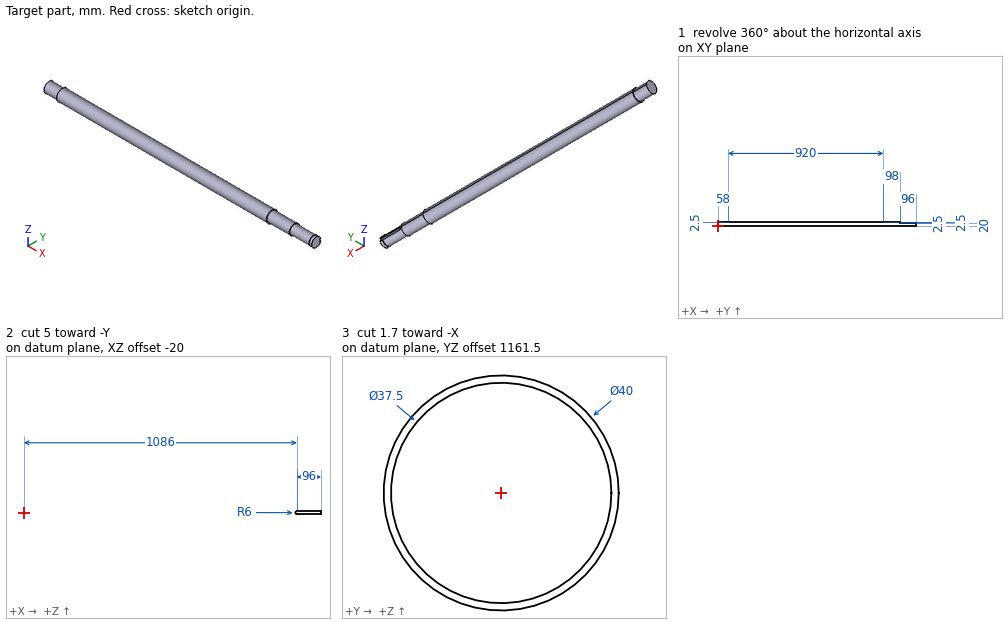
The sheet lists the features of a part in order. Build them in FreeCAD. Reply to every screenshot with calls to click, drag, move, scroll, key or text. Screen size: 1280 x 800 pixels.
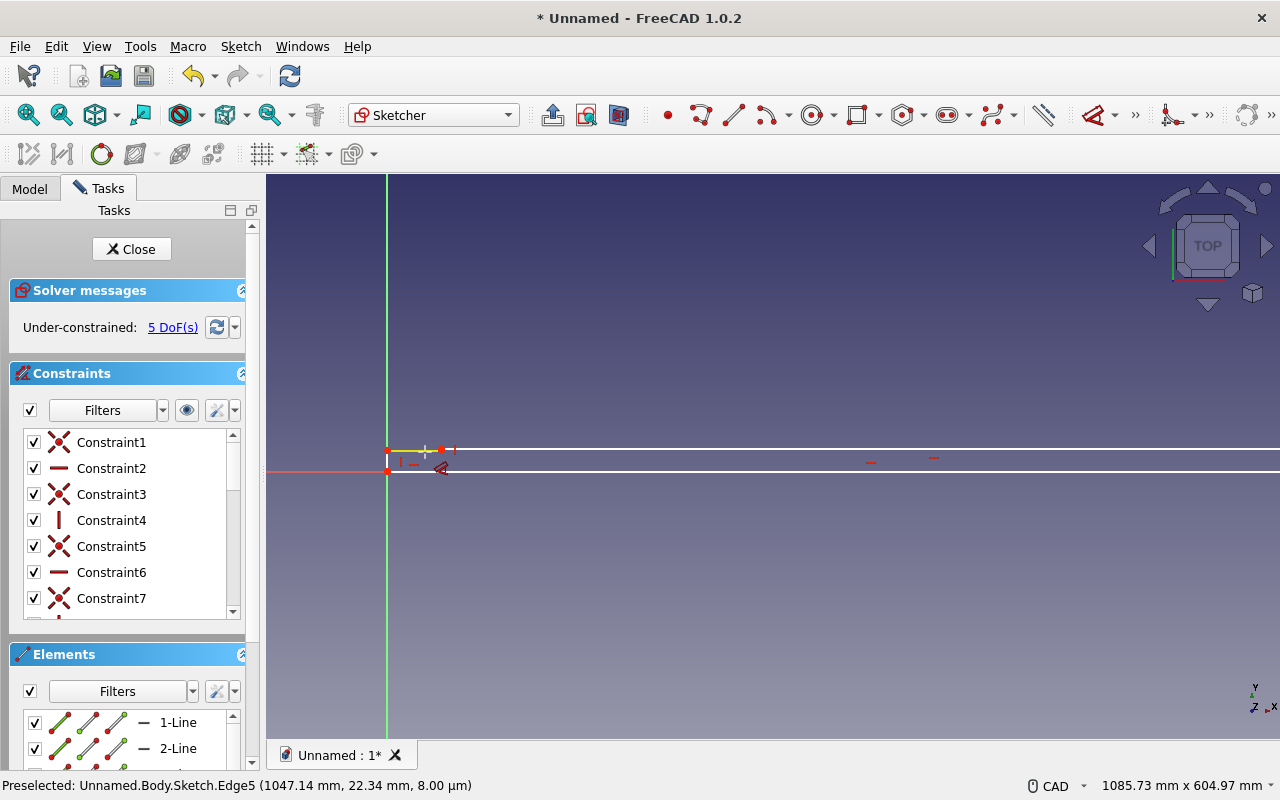
click(425, 451)
click(414, 417)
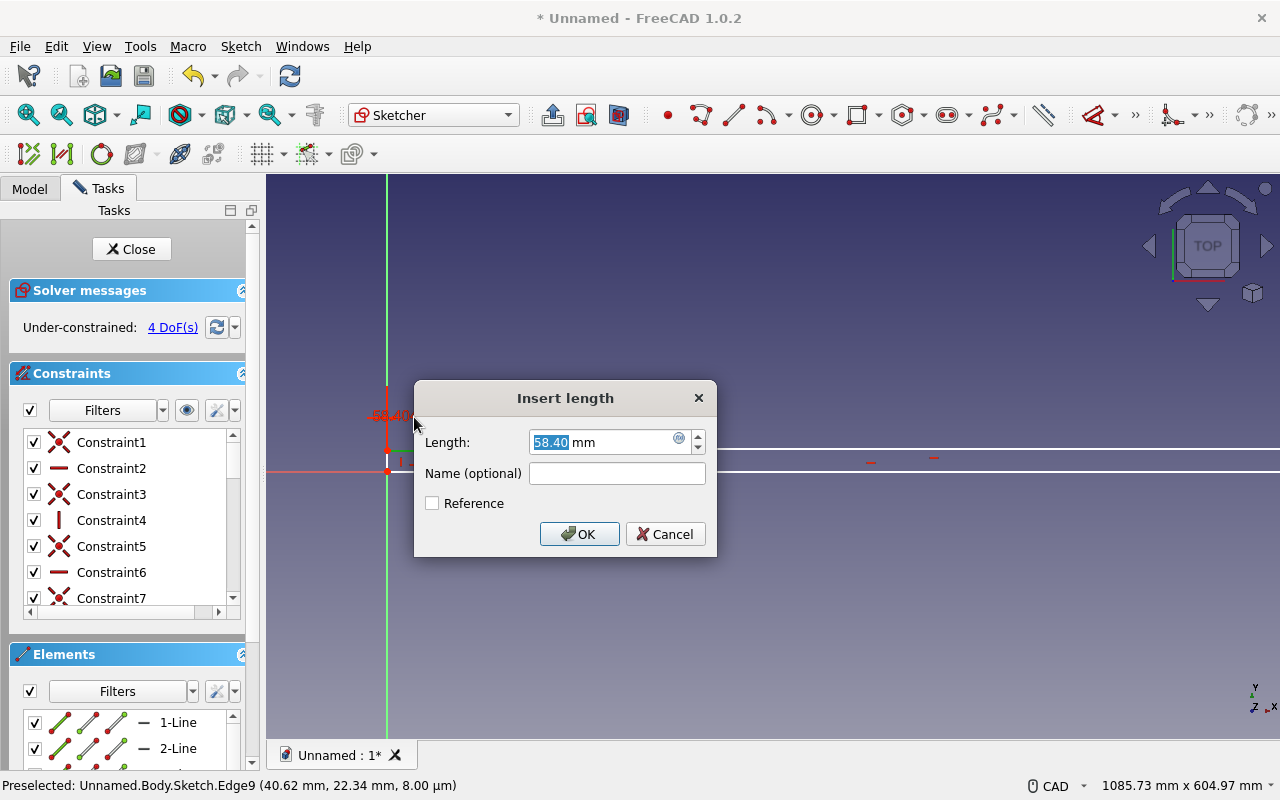
text(58)
key(Return)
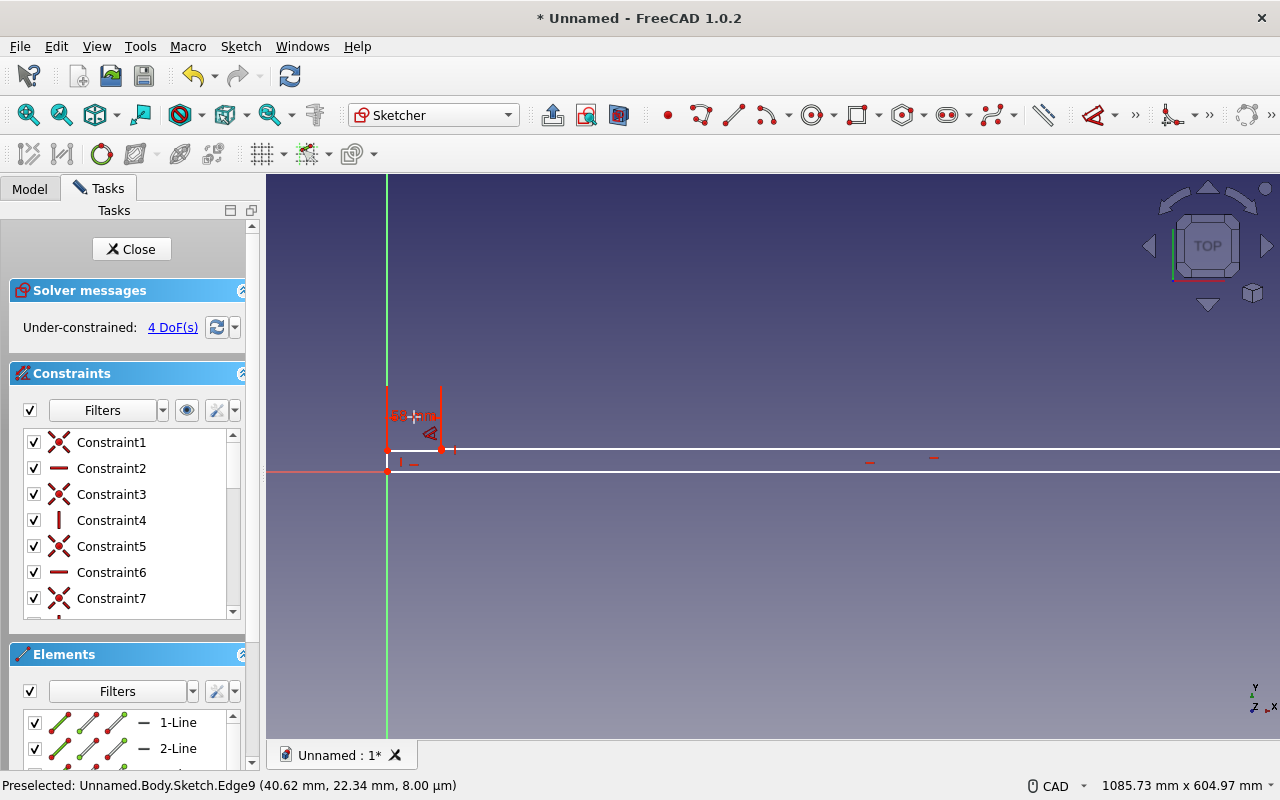
scroll(425, 452, down, 3)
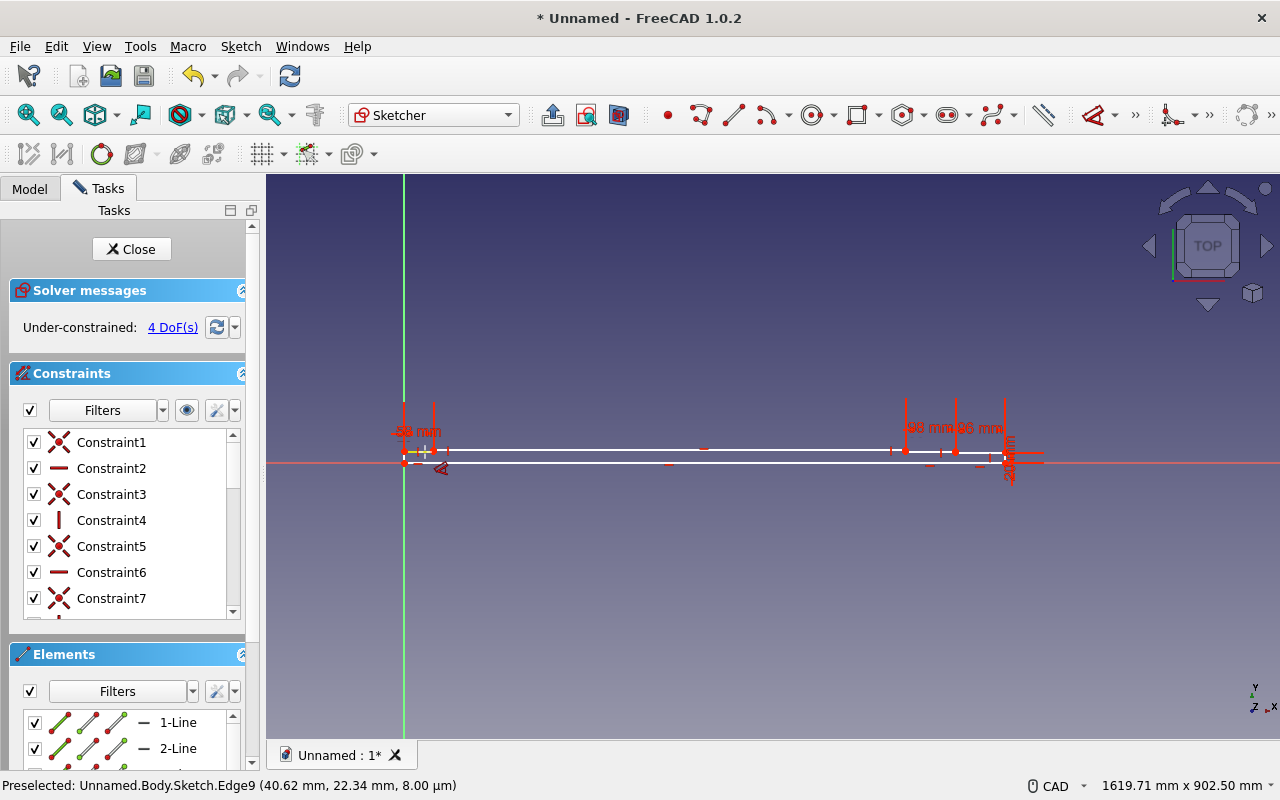
scroll(956, 452, up, 18)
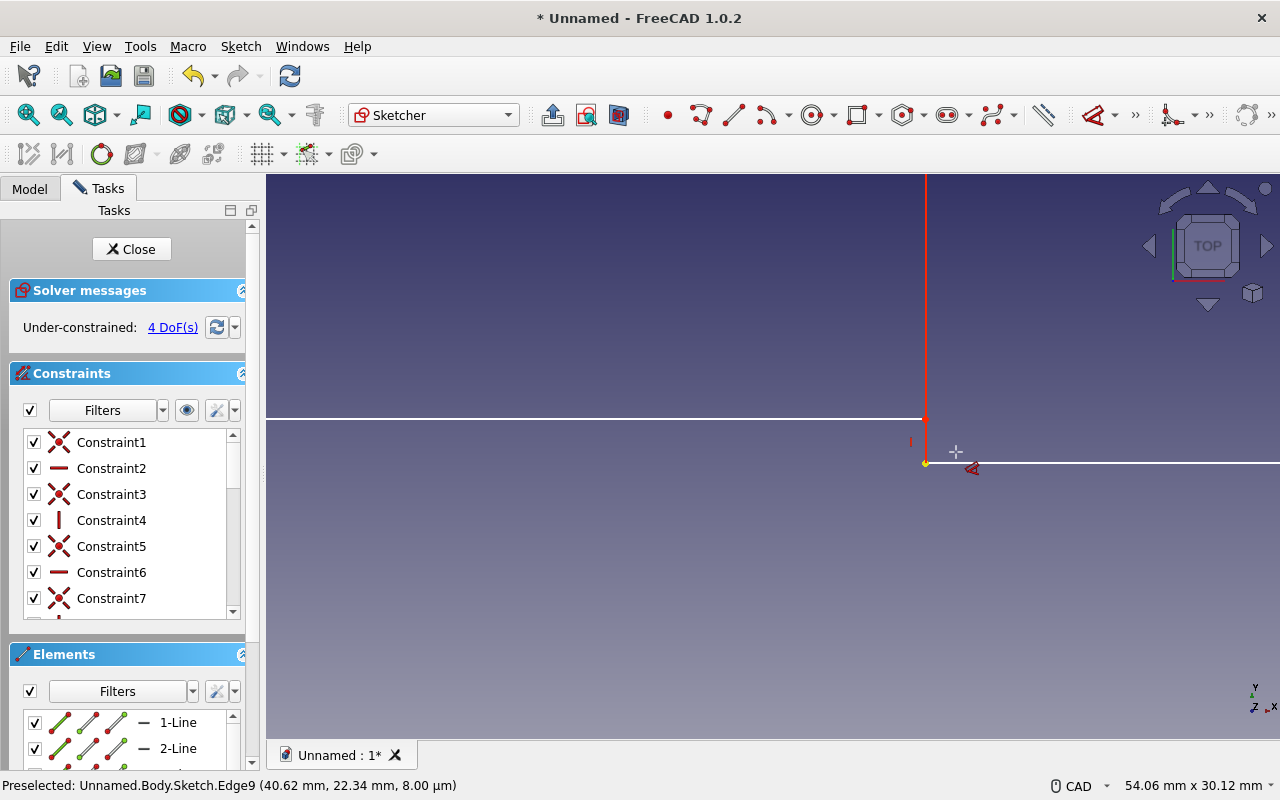
click(926, 441)
click(960, 441)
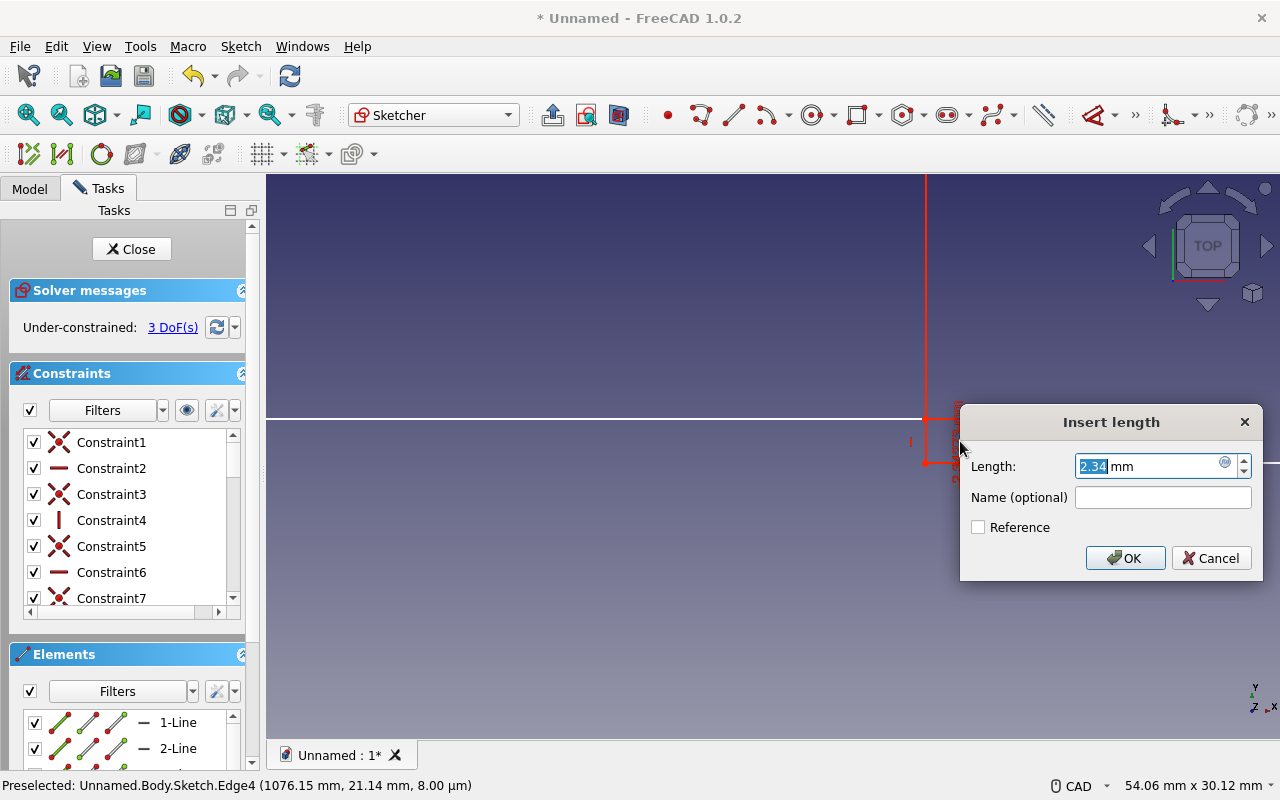
text(2.5)
key(Return)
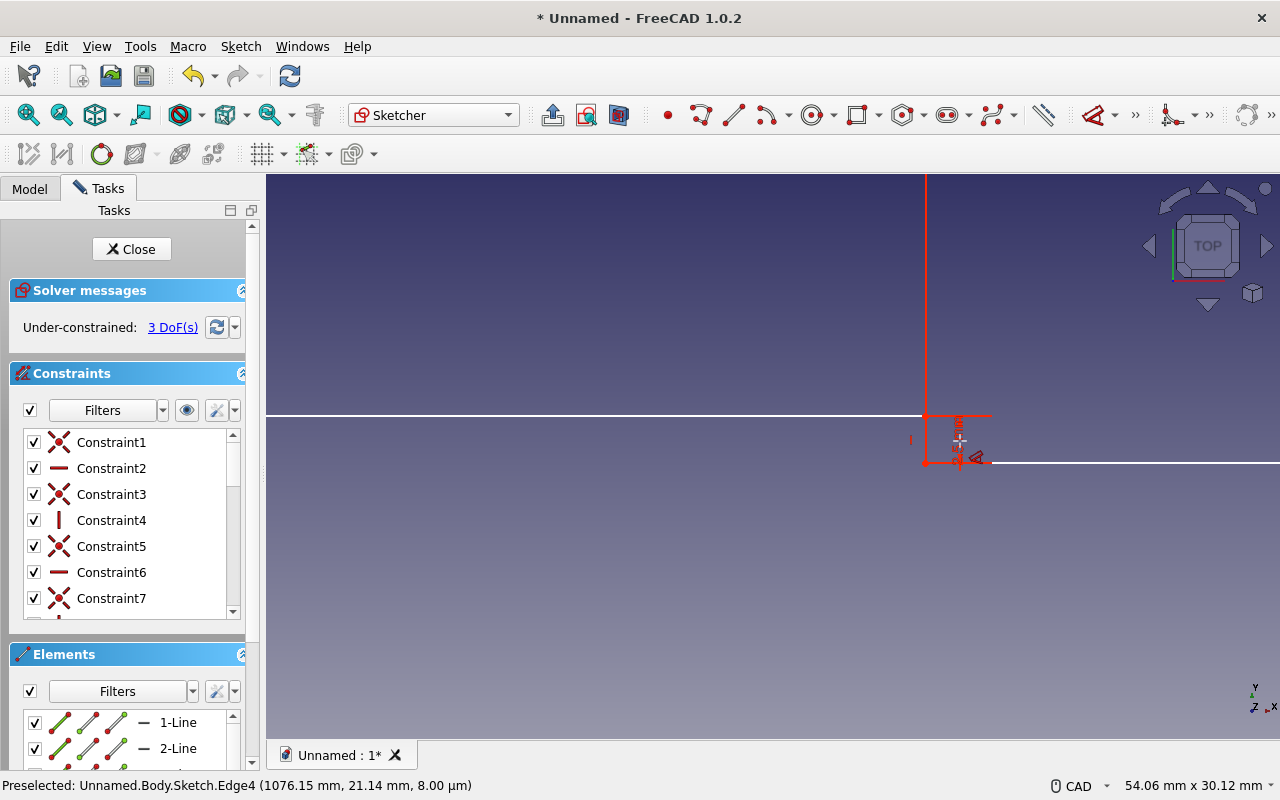
scroll(1014, 451, down, 17)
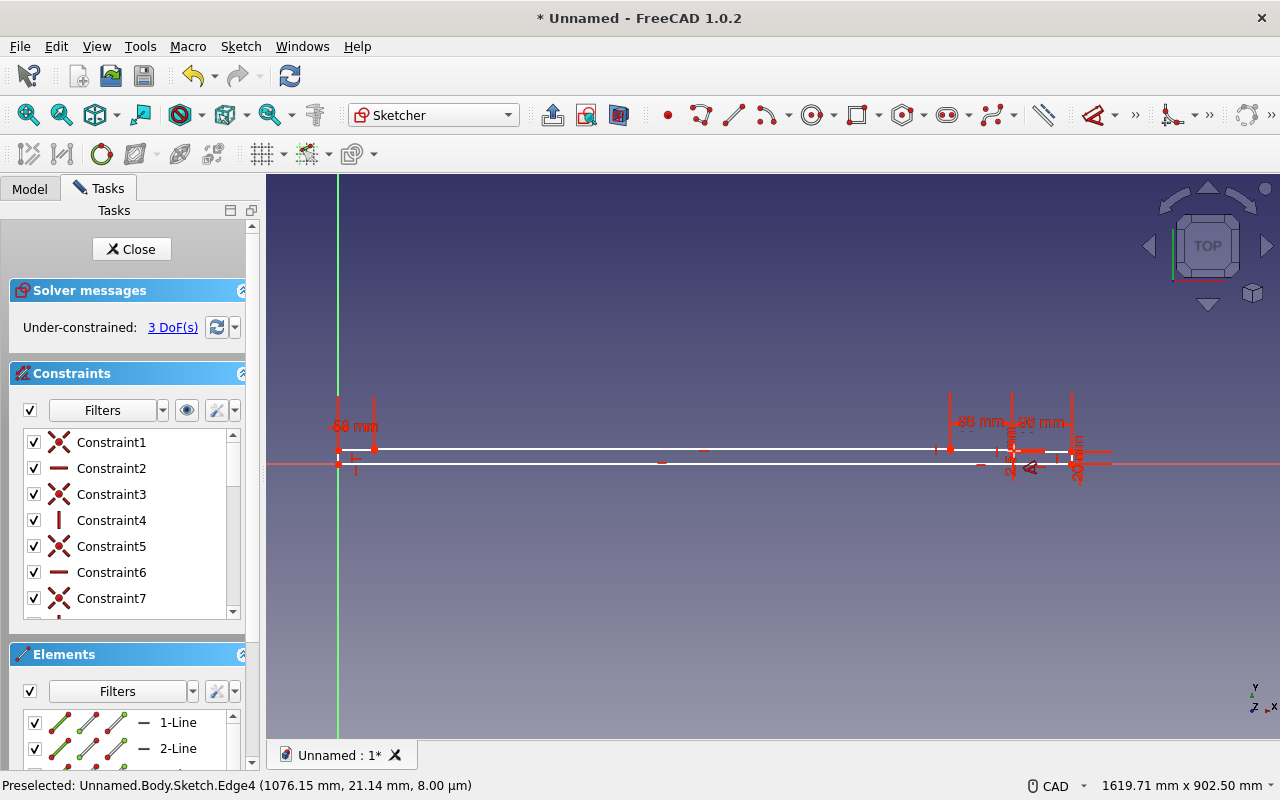
scroll(950, 450, up, 17)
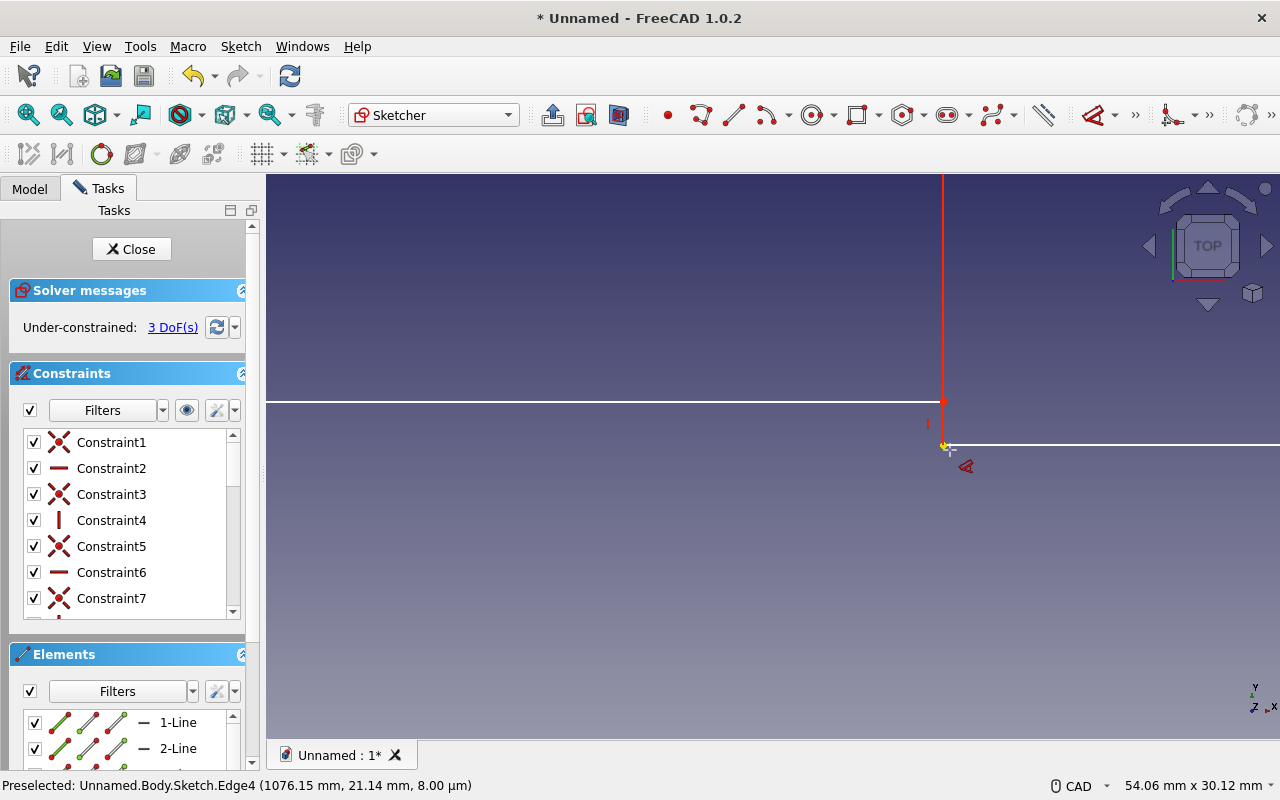
click(943, 432)
click(977, 424)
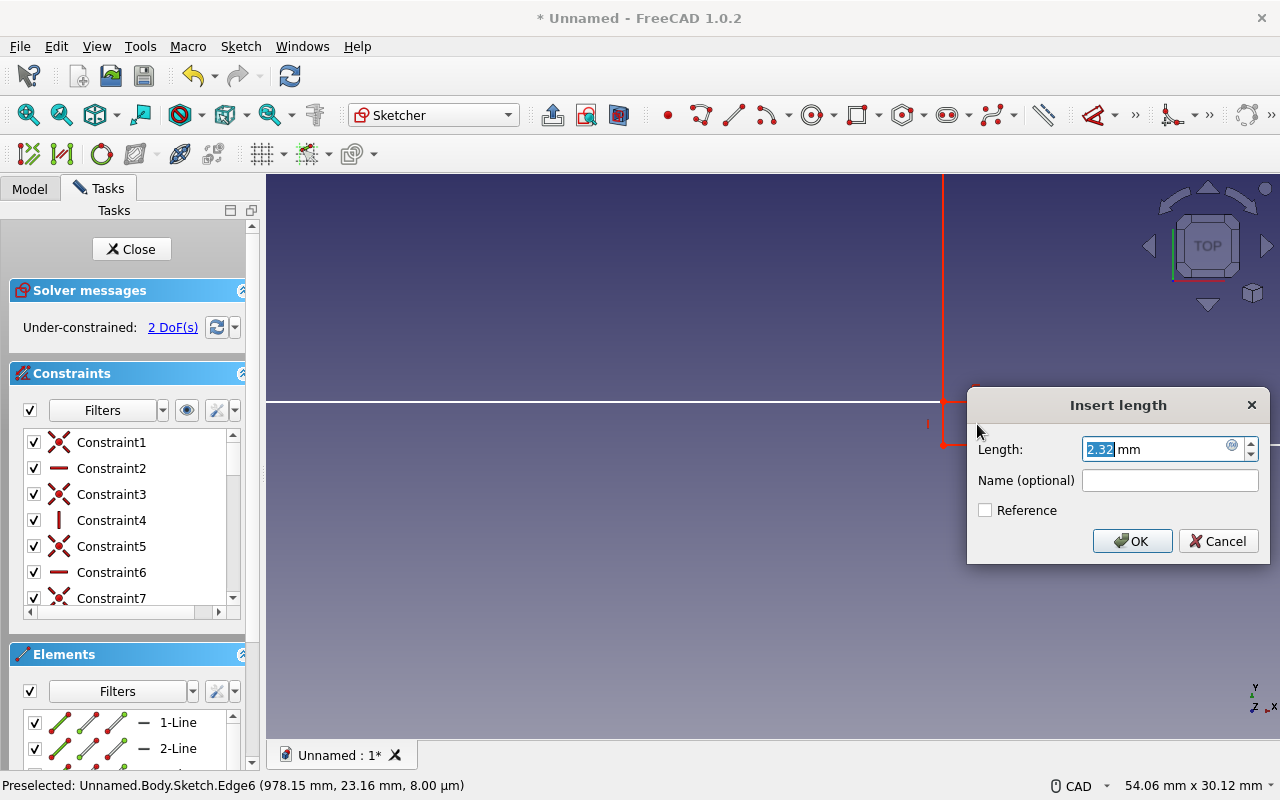
text(2.5)
key(Return)